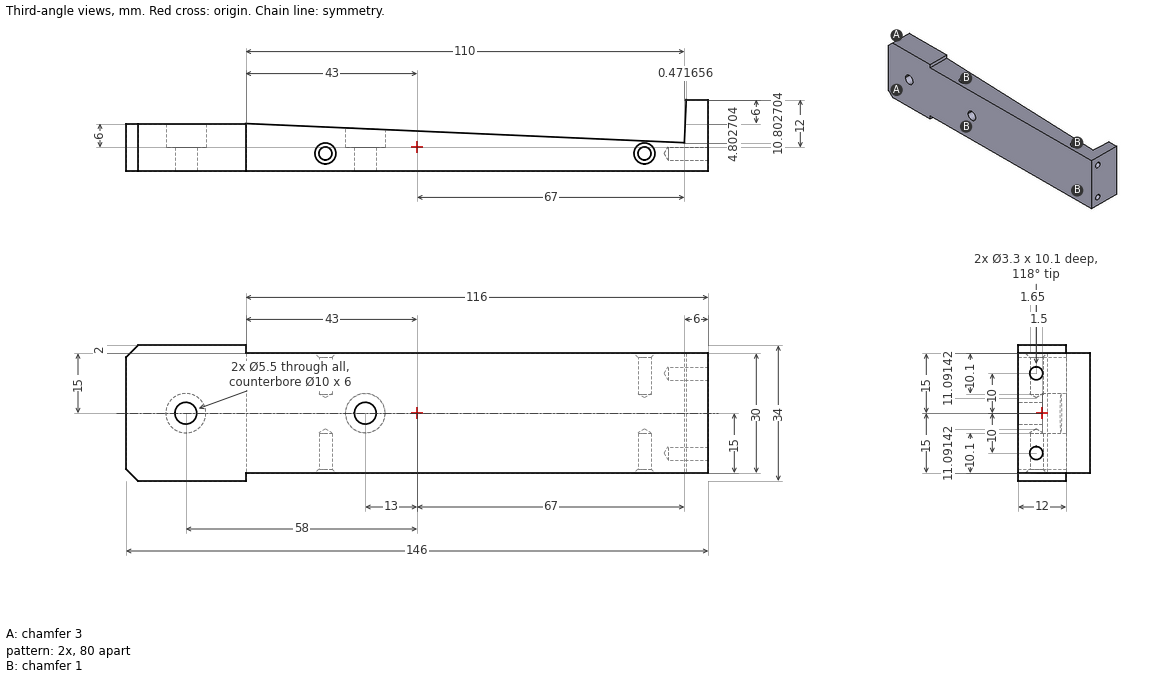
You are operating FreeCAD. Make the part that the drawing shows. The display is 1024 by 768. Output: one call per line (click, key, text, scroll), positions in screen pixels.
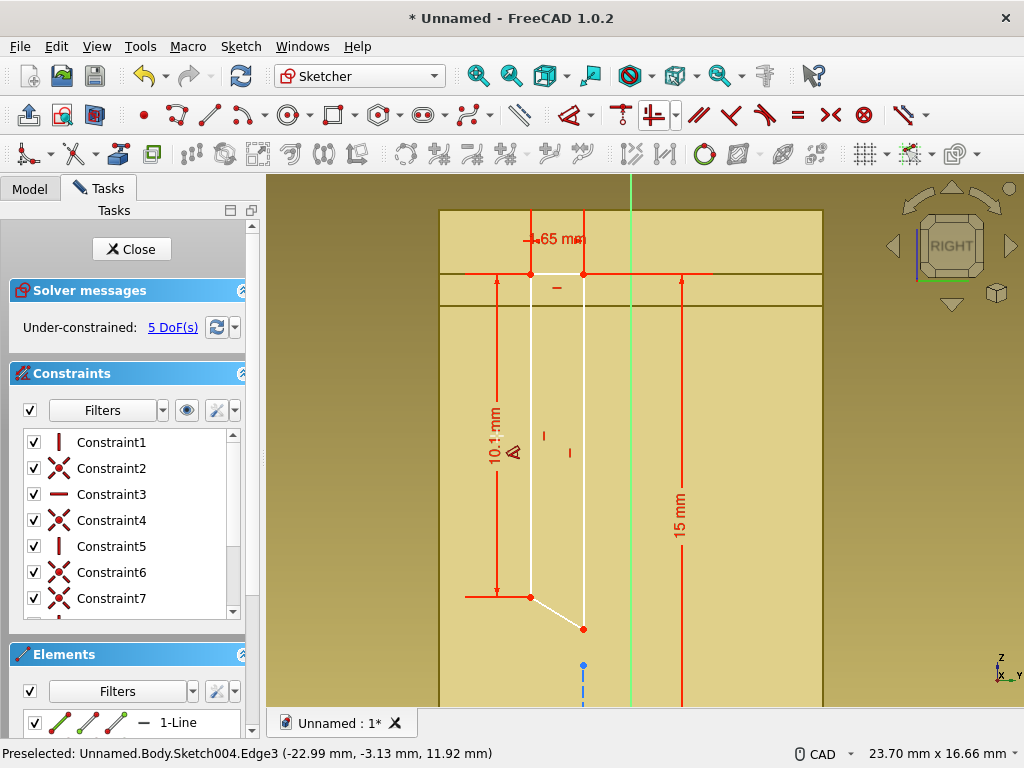
click(584, 630)
click(607, 596)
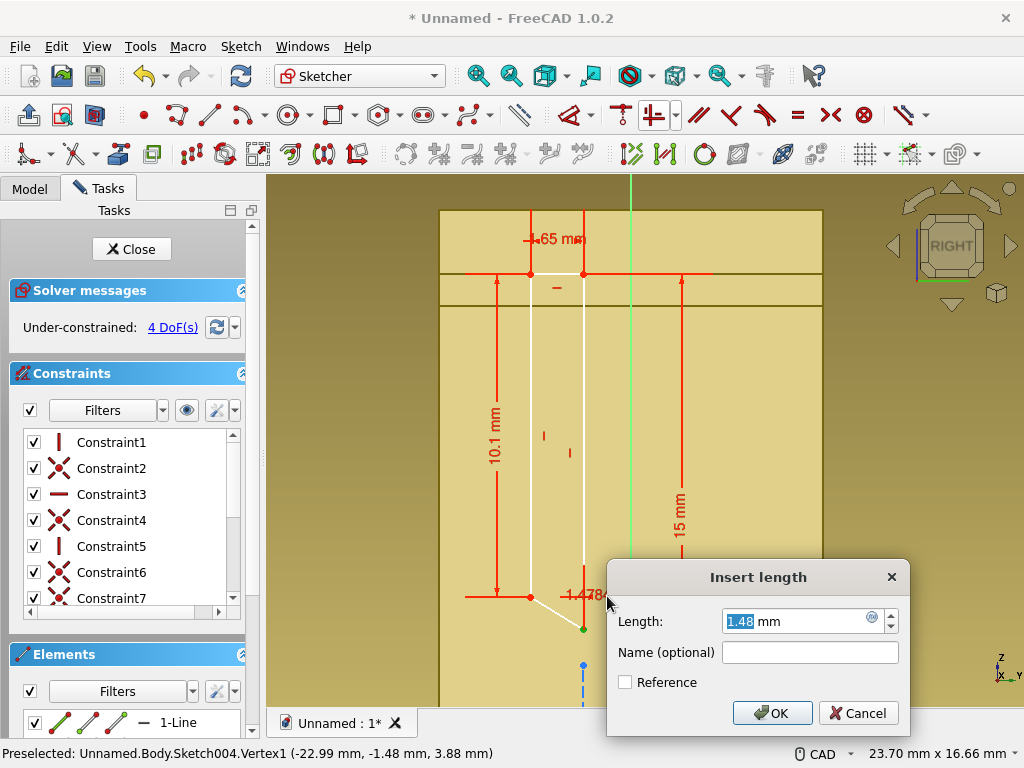
text(1.5)
key(Return)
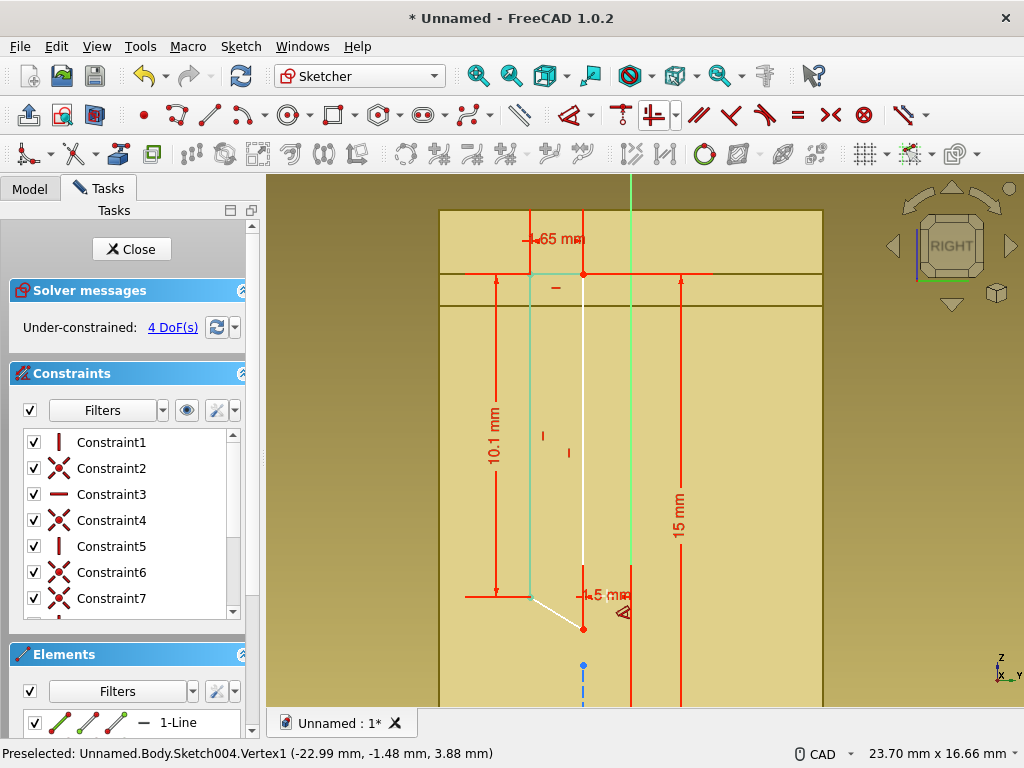
click(583, 666)
click(607, 632)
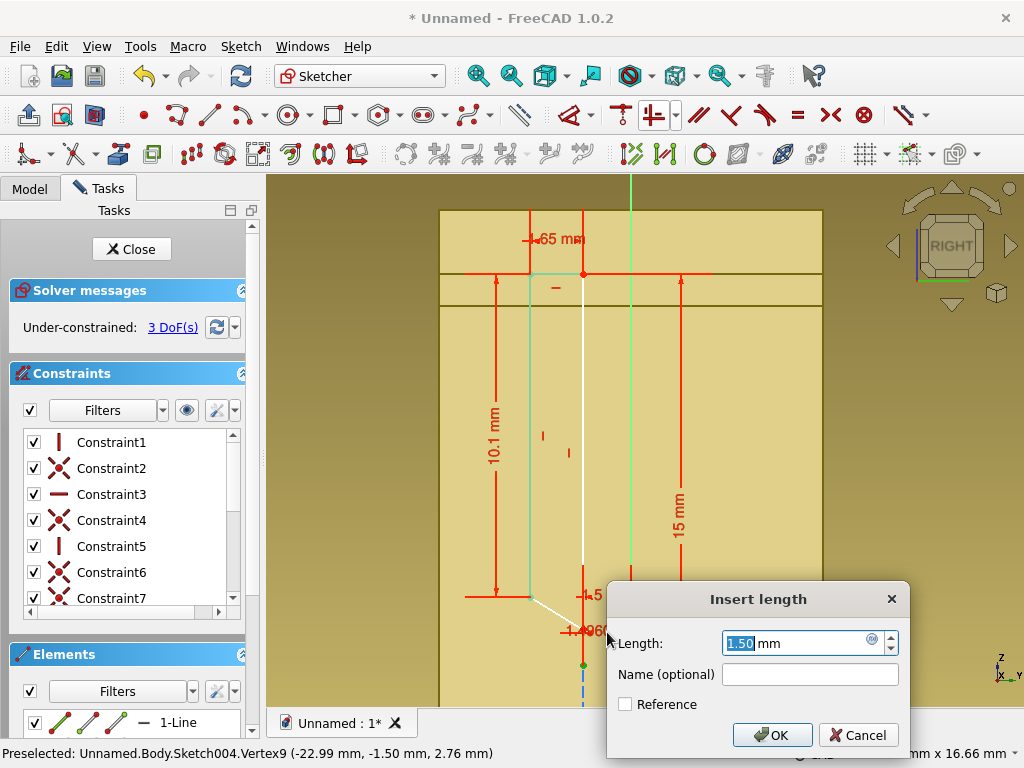
text(1.5)
key(Return)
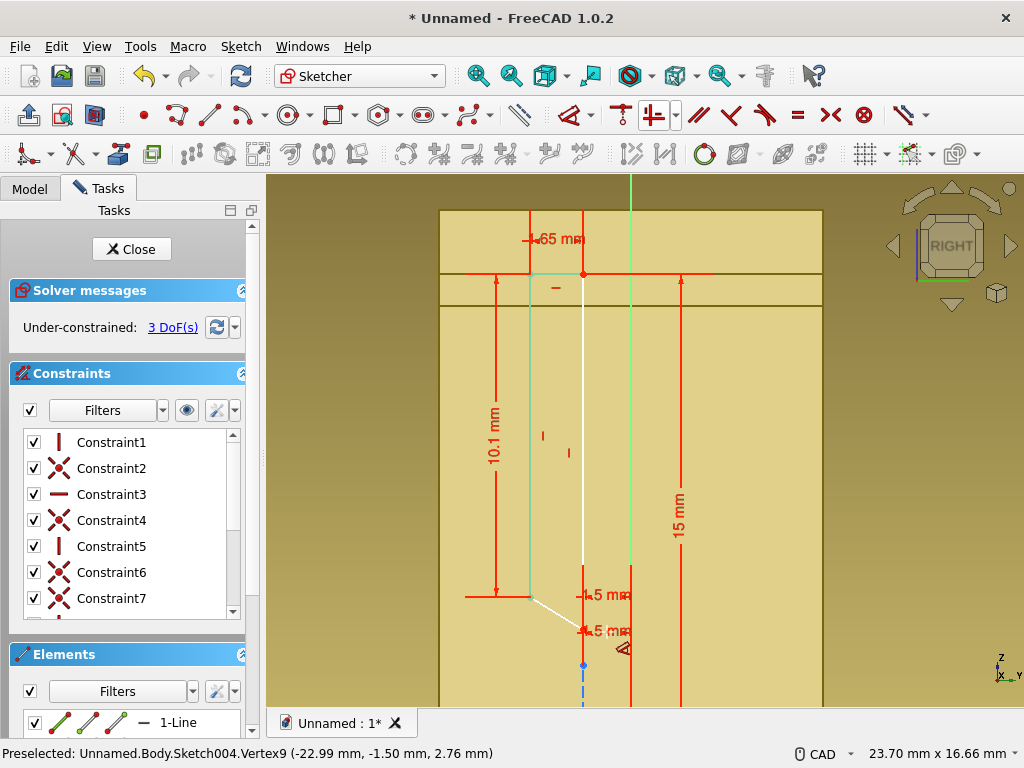
click(583, 523)
click(617, 452)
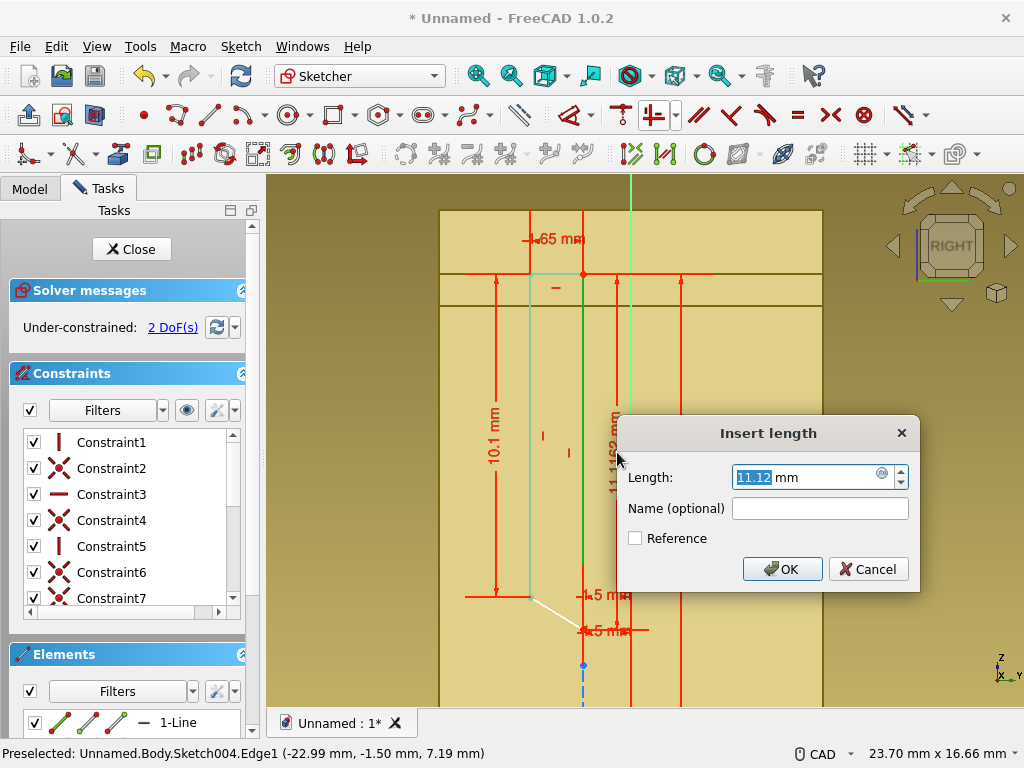
text(11.09142)
key(Return)
key(Escape)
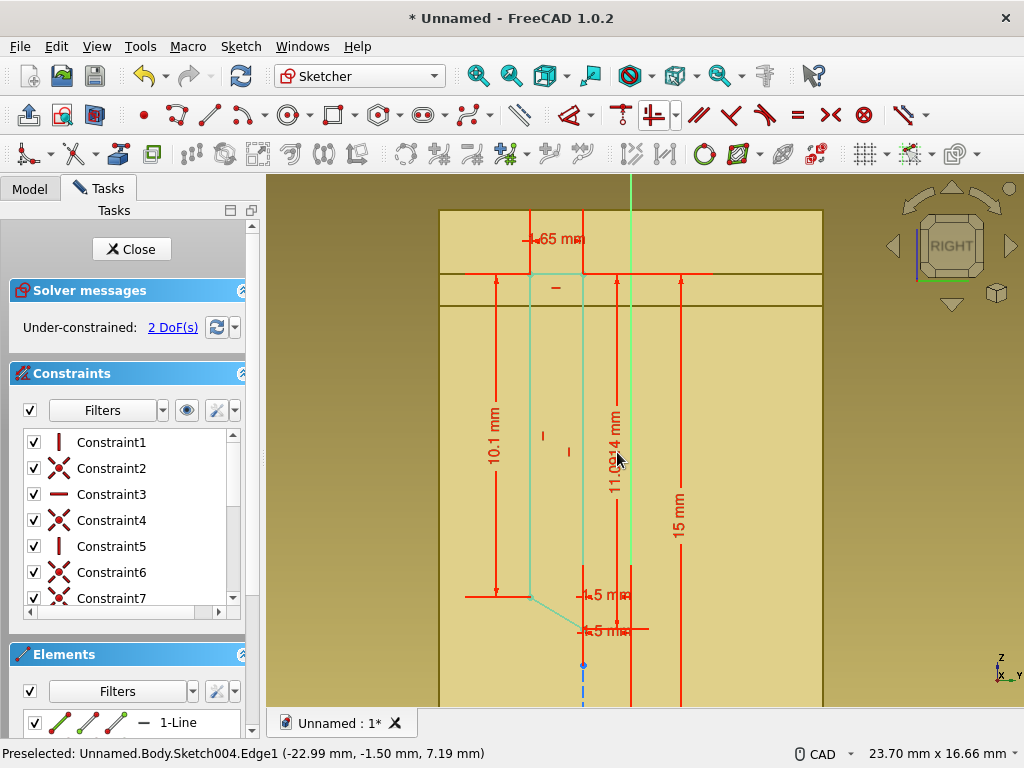
click(132, 249)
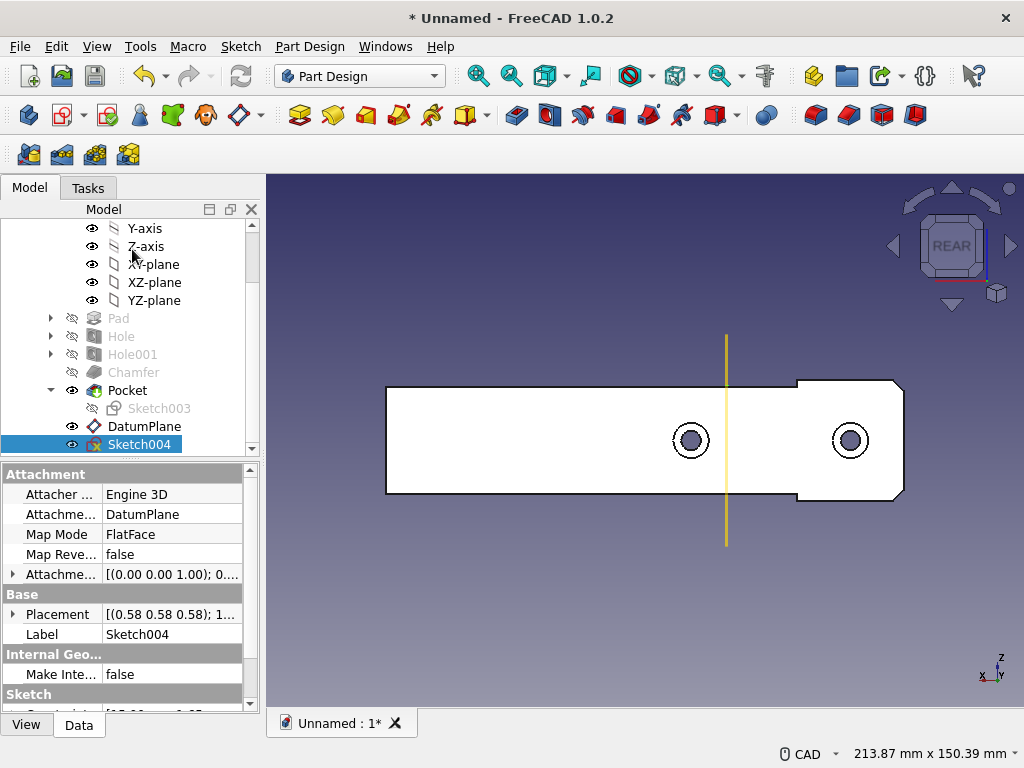
click(583, 116)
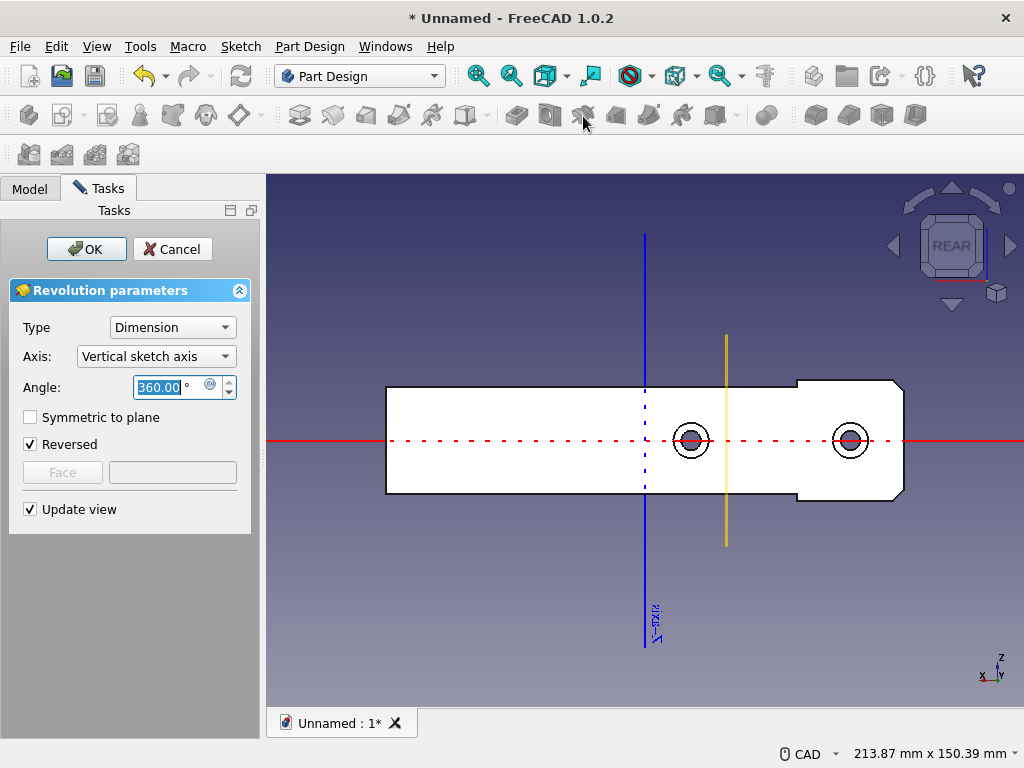
click(157, 356)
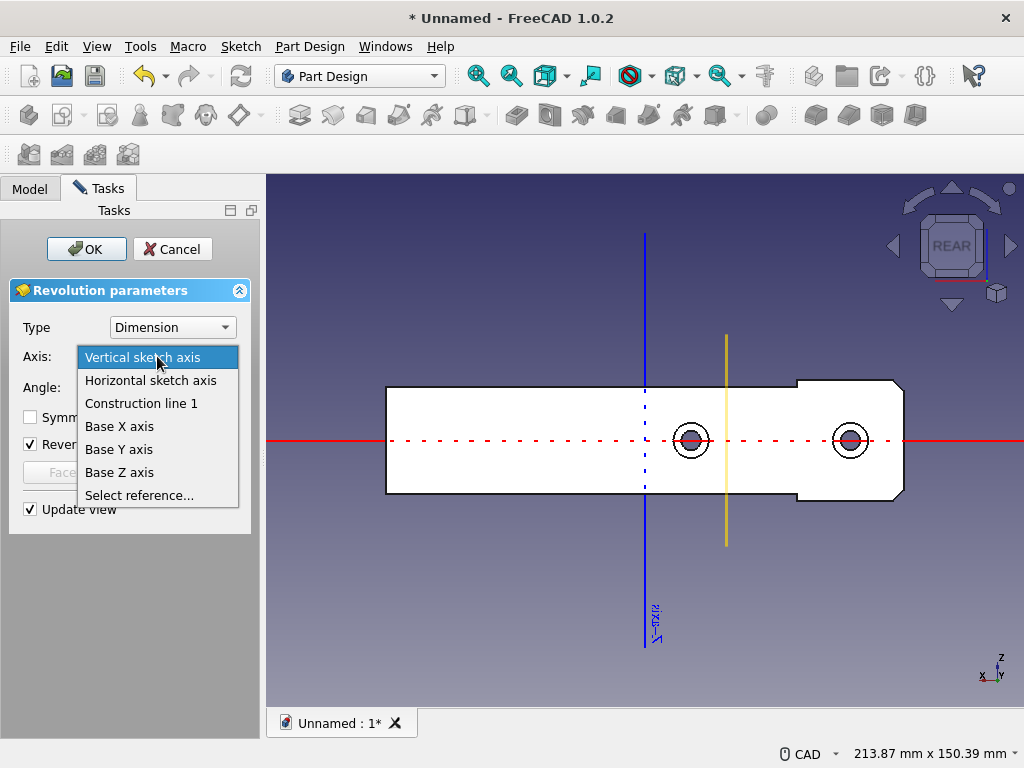
click(156, 404)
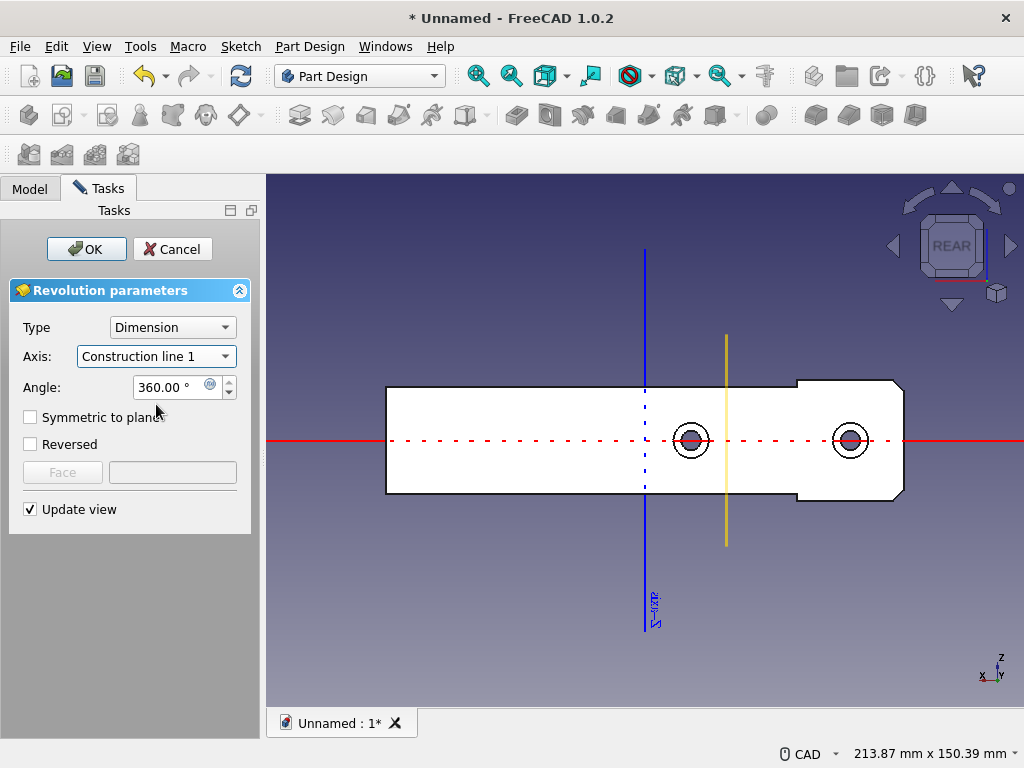
click(87, 249)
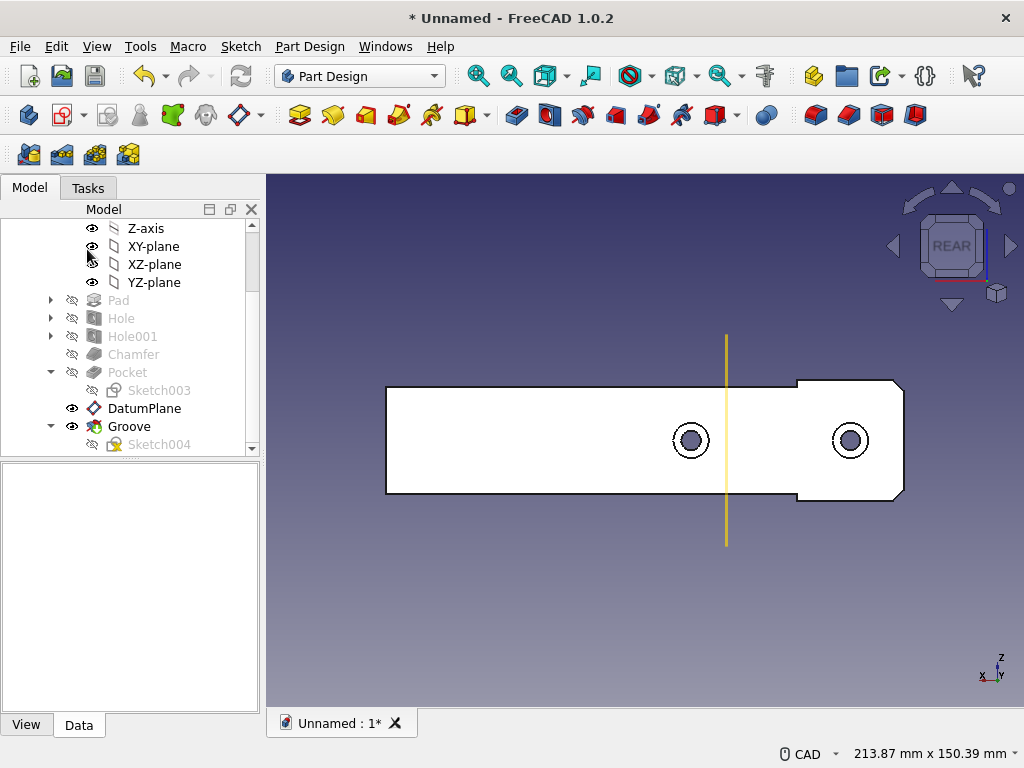
click(117, 408)
key(space)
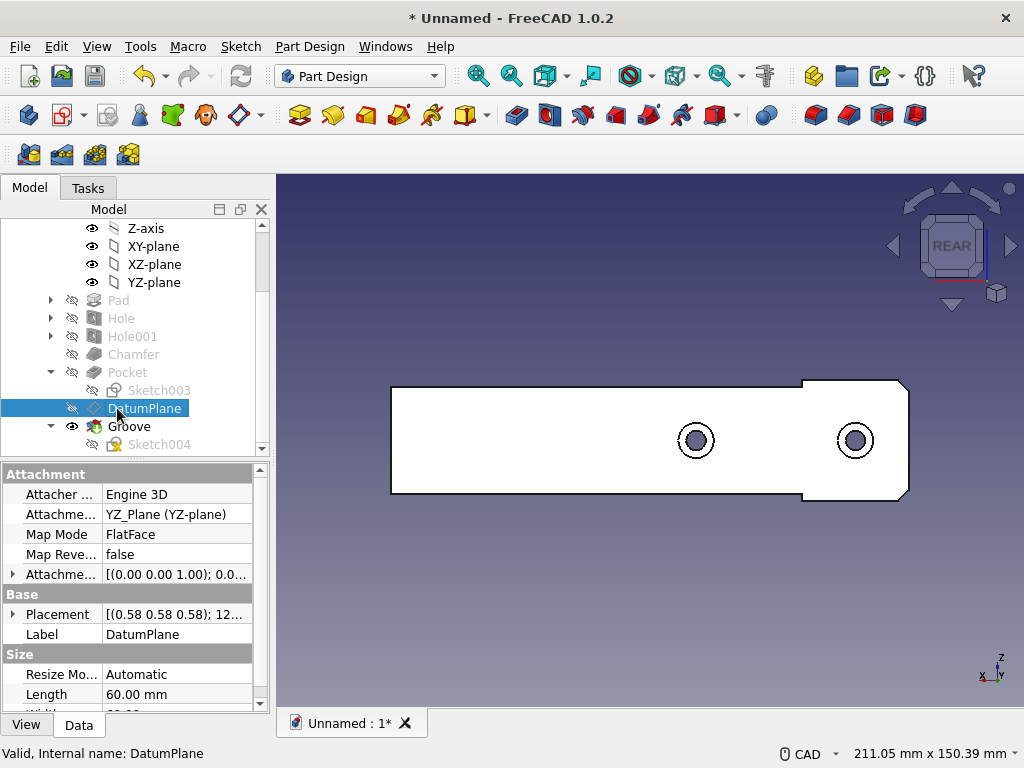
click(117, 426)